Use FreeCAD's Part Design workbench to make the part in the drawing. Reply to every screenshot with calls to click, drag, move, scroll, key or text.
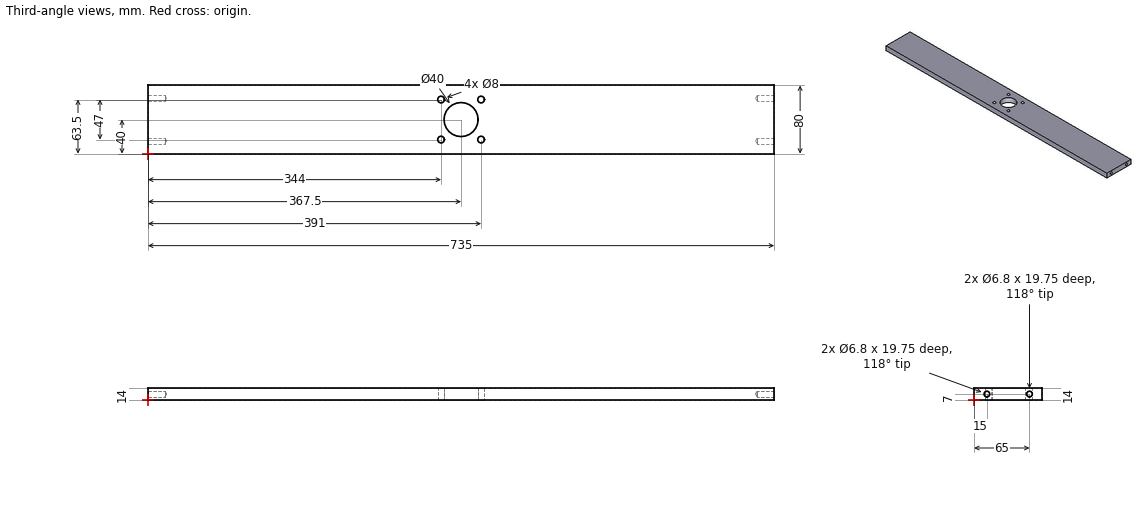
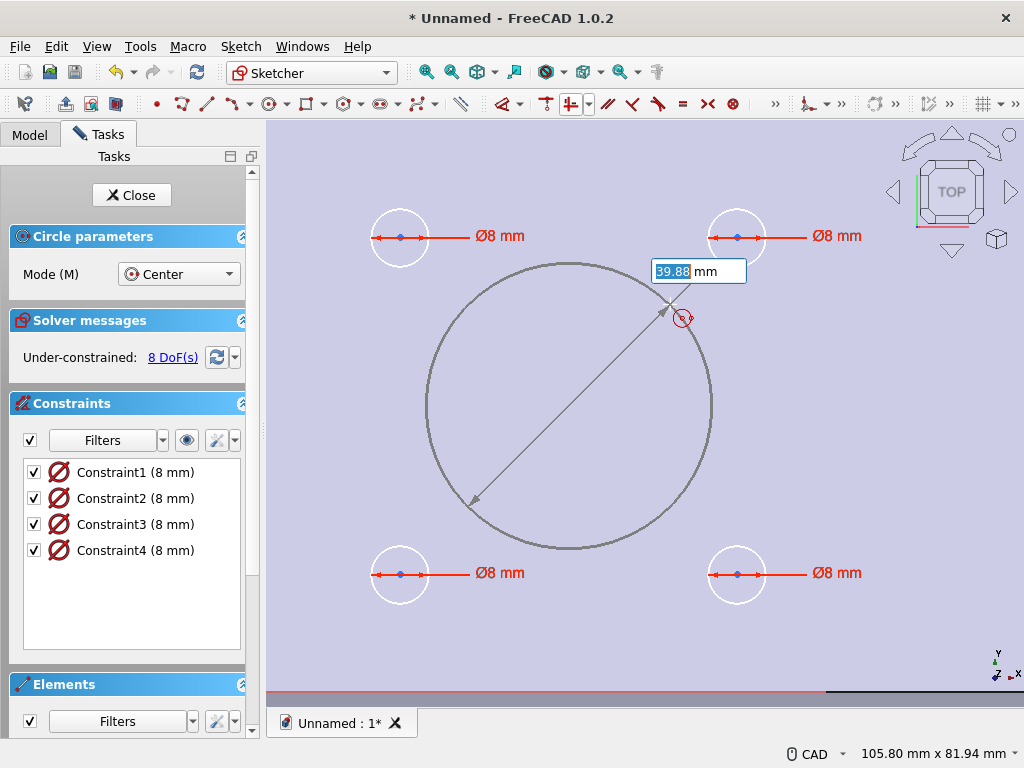
text(40)
key(Return)
key(Escape)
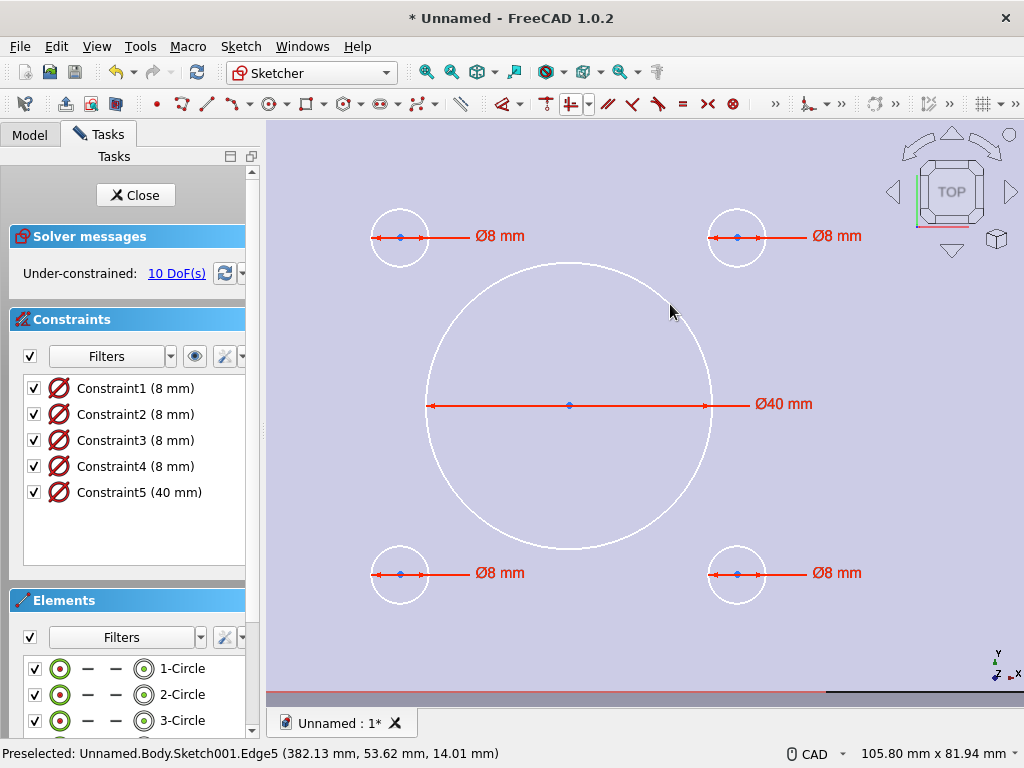
click(400, 238)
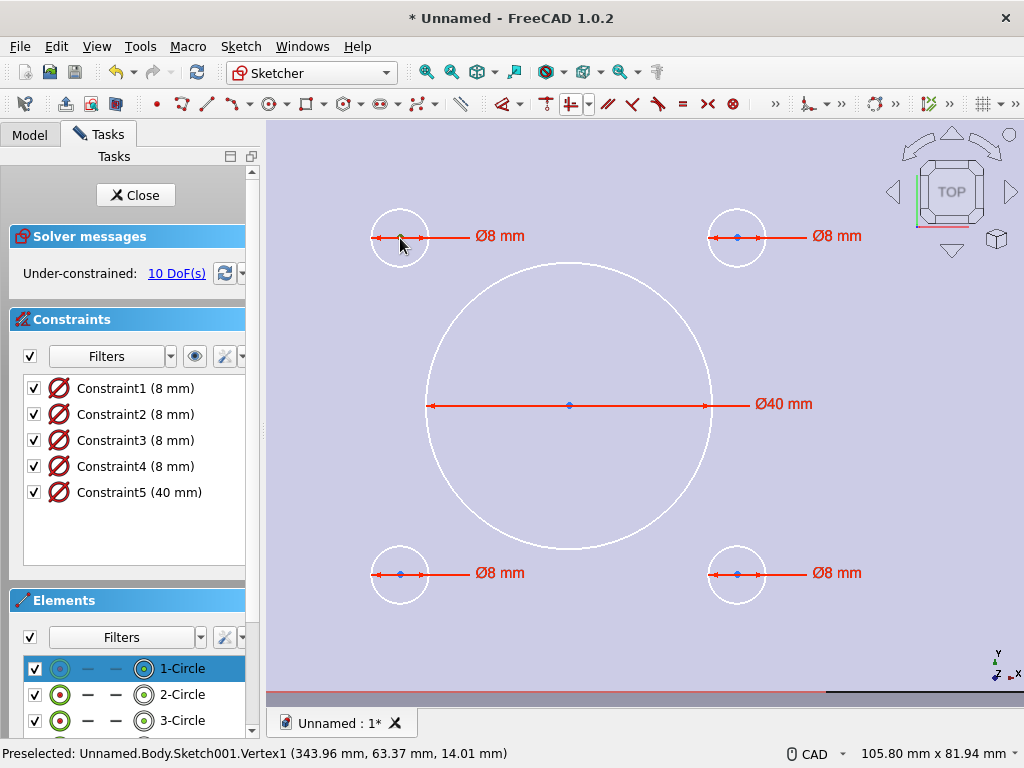
click(400, 575)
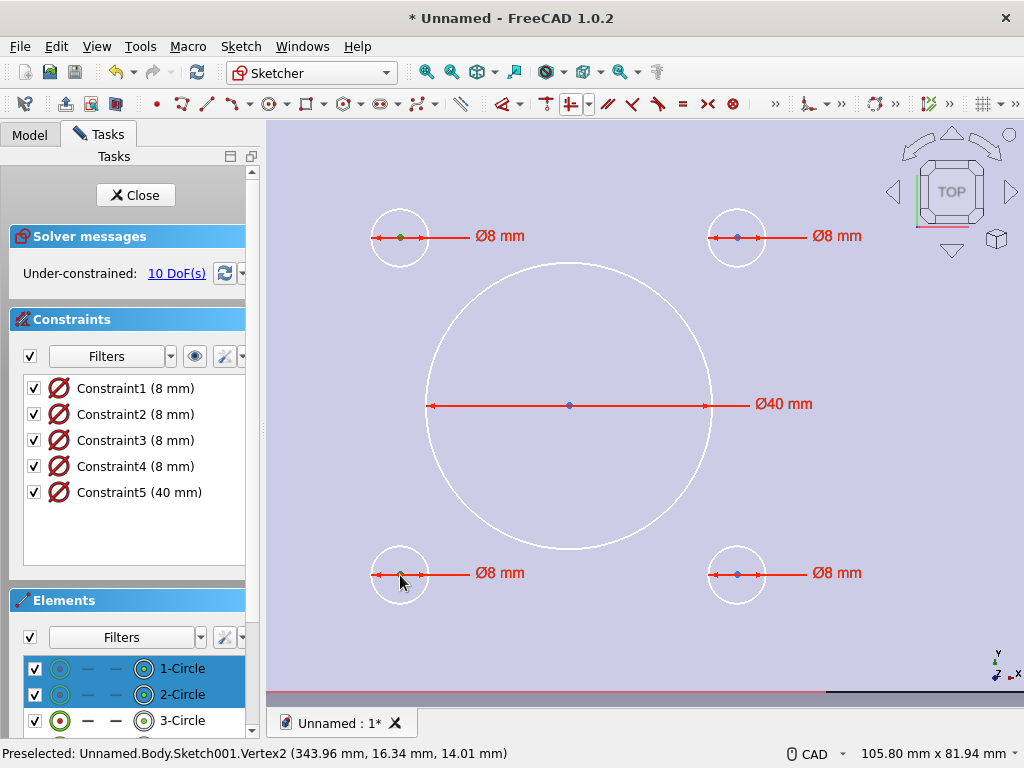
key(v)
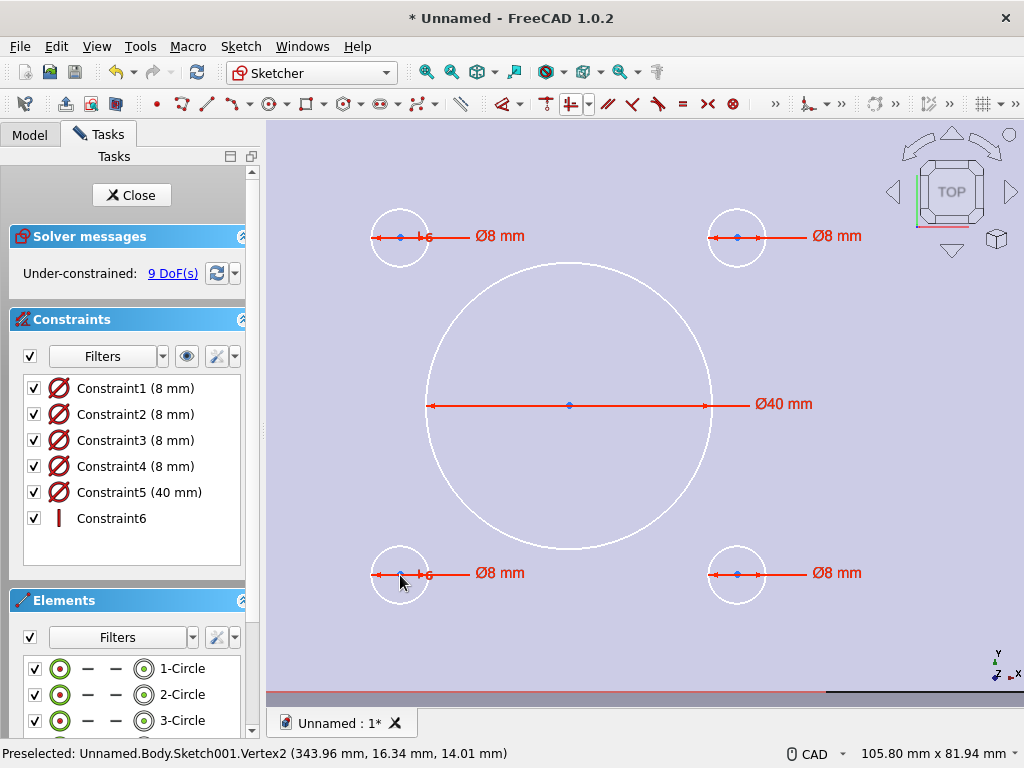
click(400, 575)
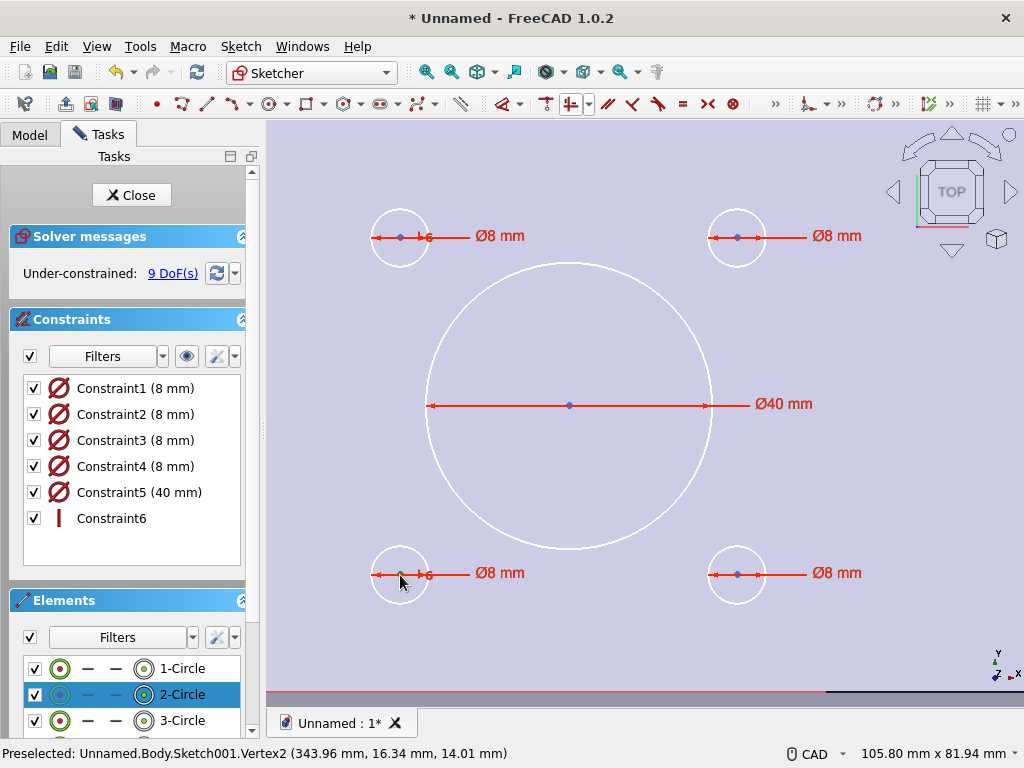
click(737, 575)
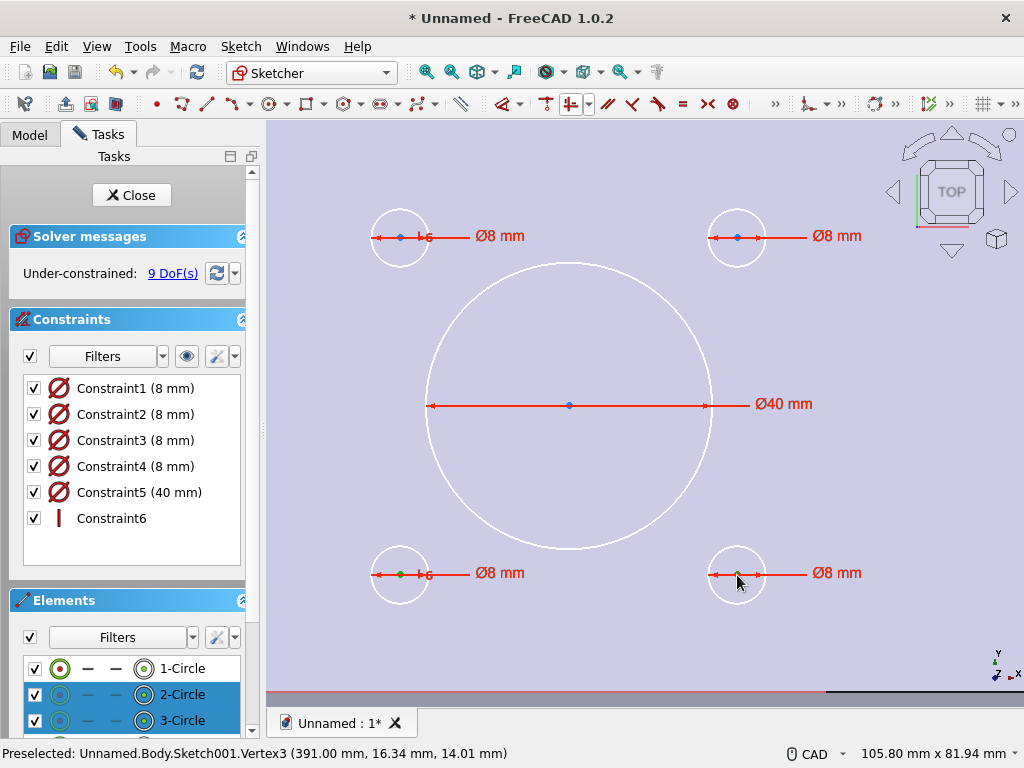
key(h)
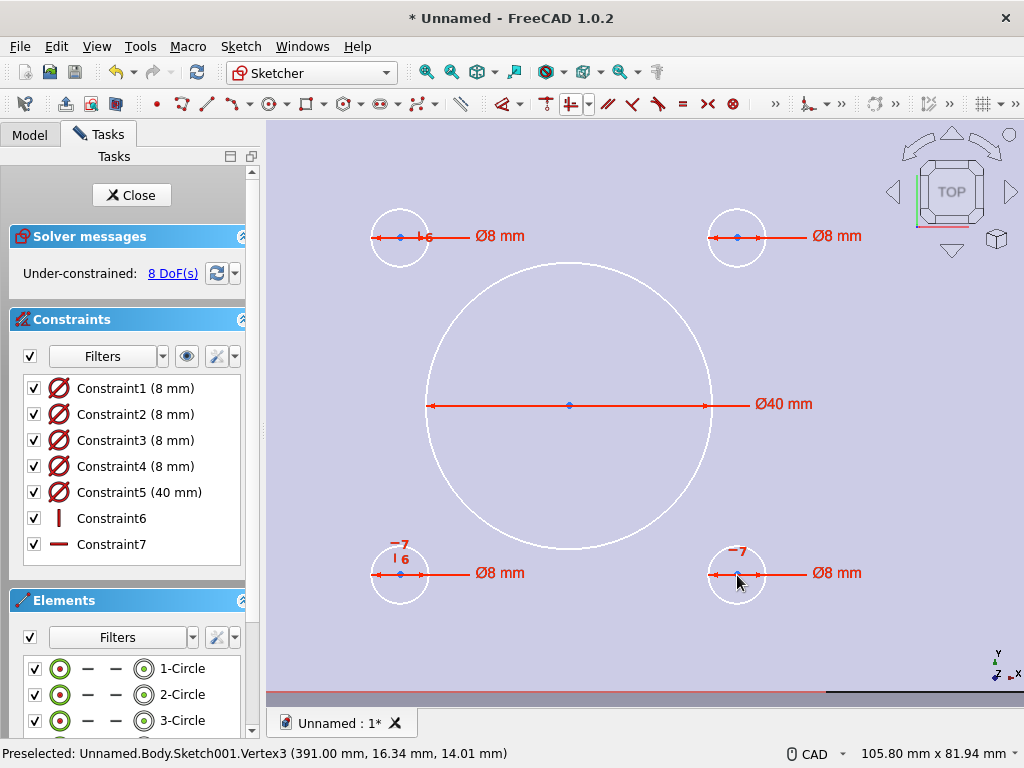
click(737, 575)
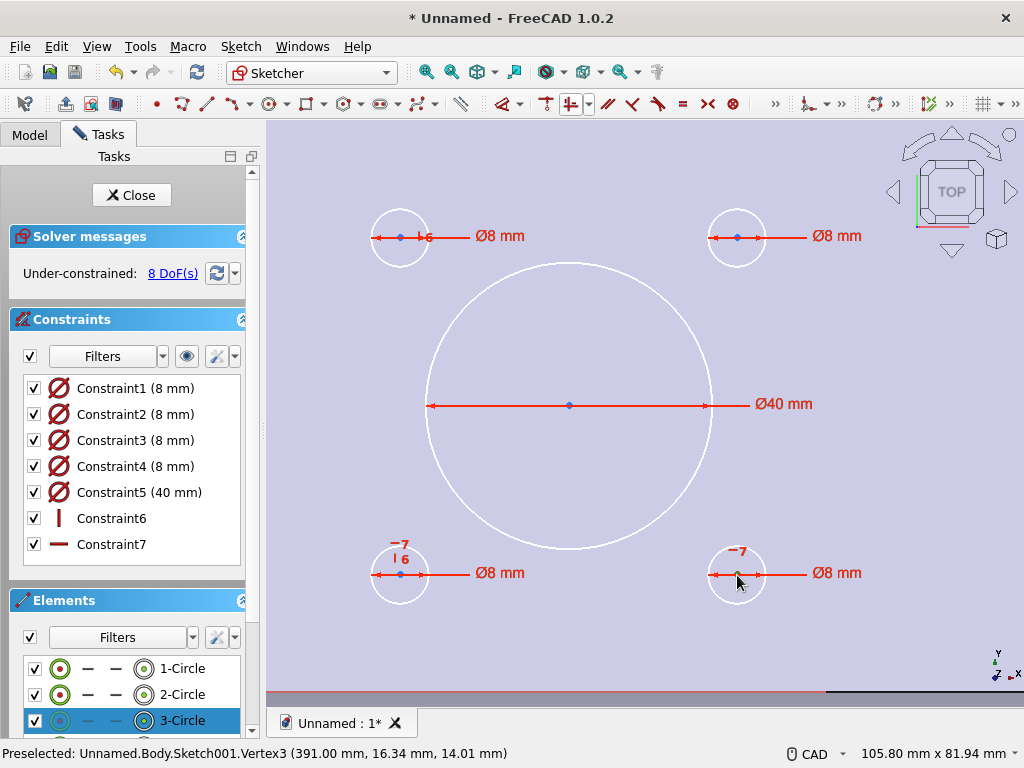
click(737, 238)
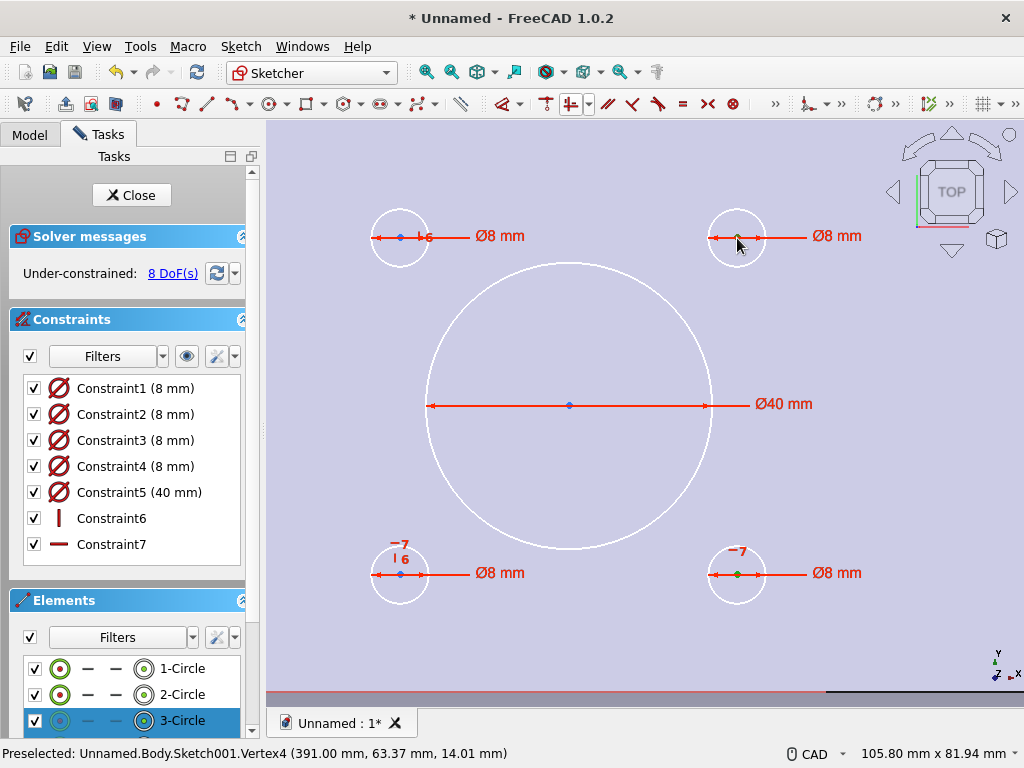
key(v)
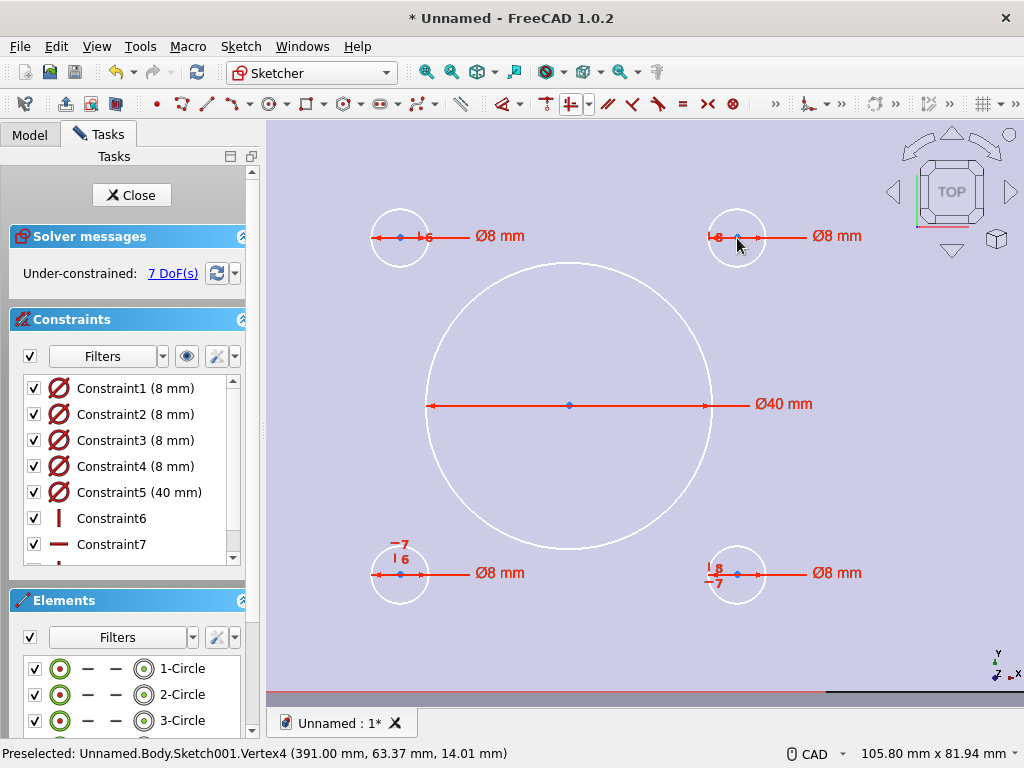
click(400, 238)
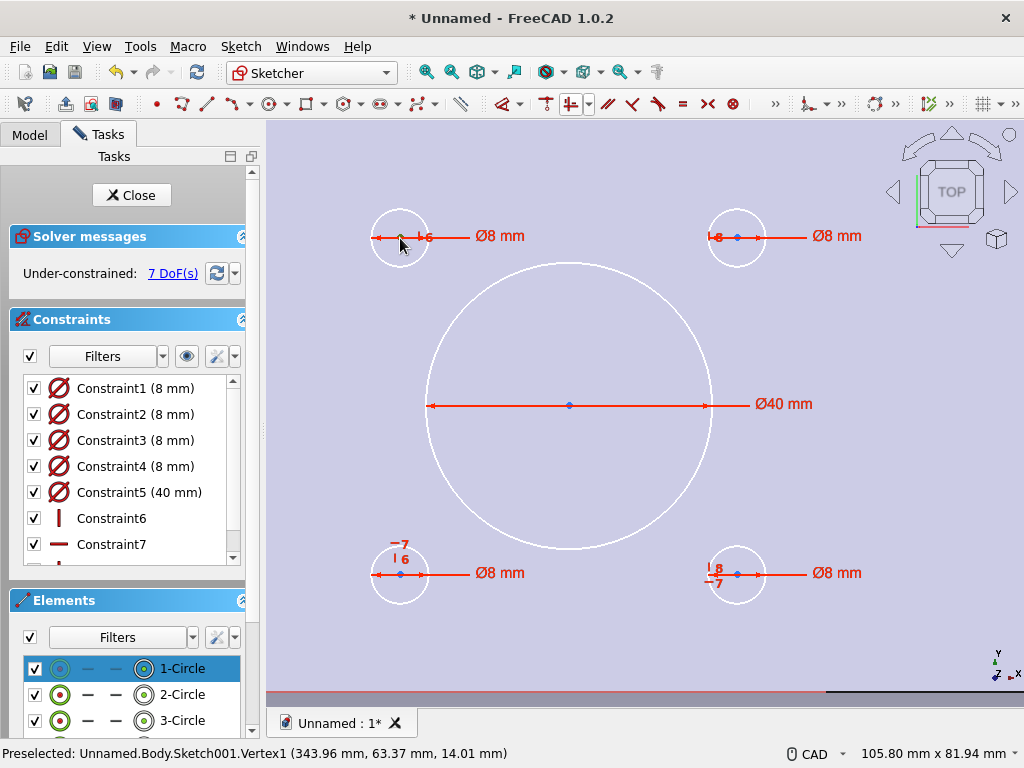
click(737, 238)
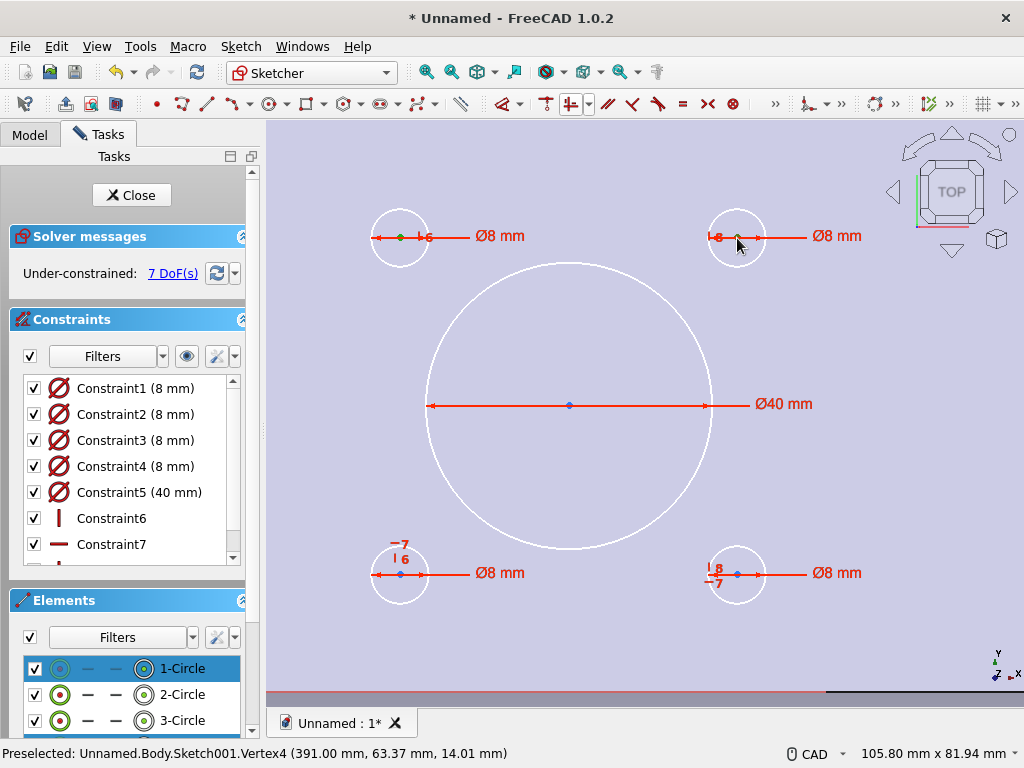
key(h)